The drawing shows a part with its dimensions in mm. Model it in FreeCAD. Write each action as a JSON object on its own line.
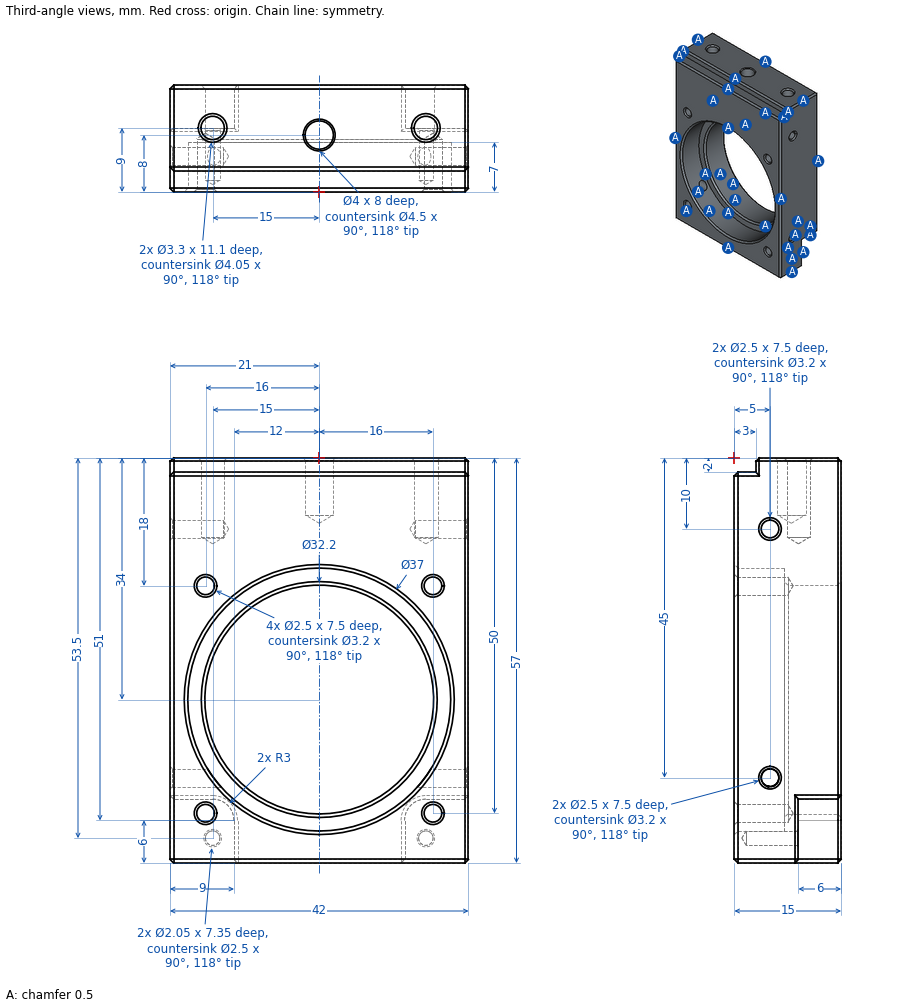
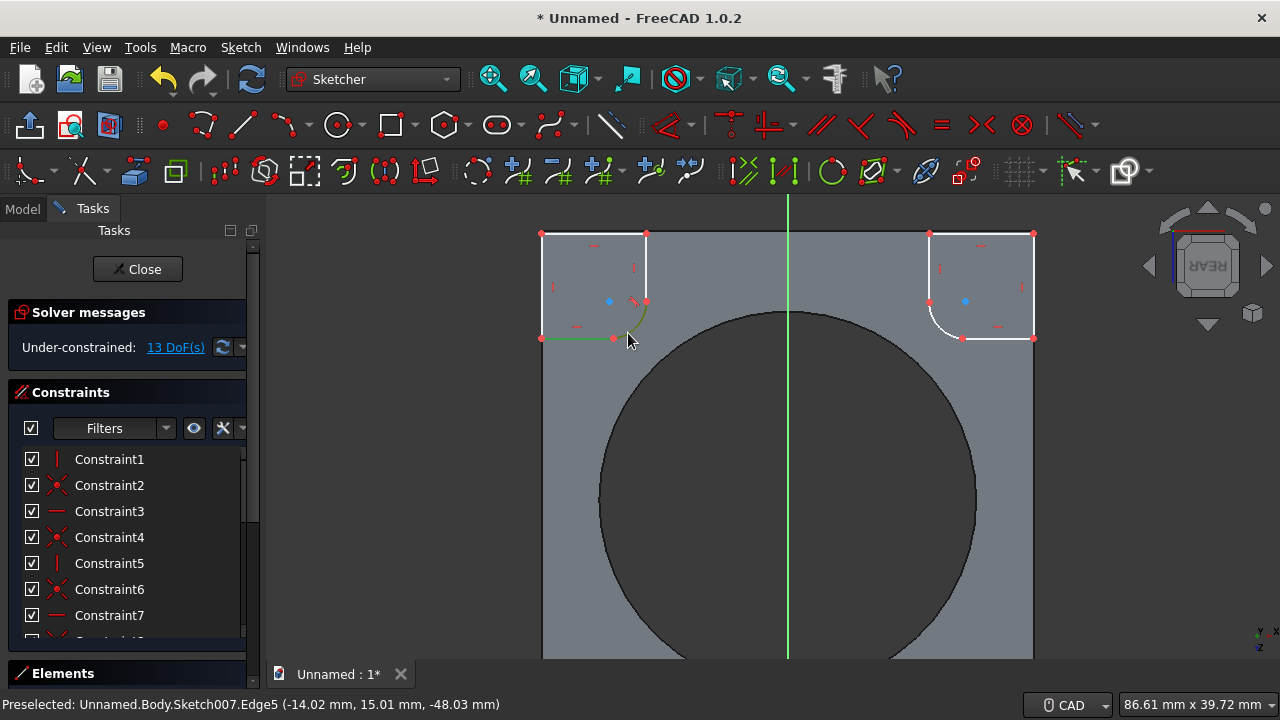
{"action": "left_click", "coordinate": [902, 126]}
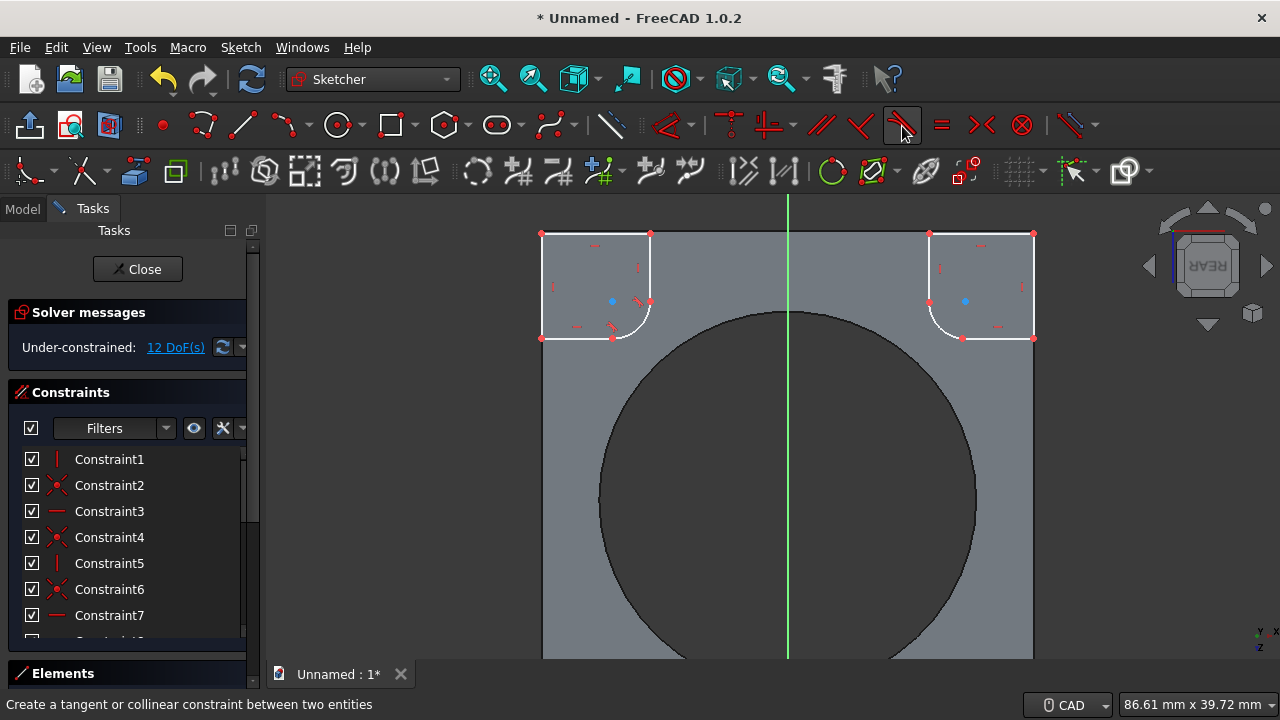
{"action": "left_click", "coordinate": [984, 339]}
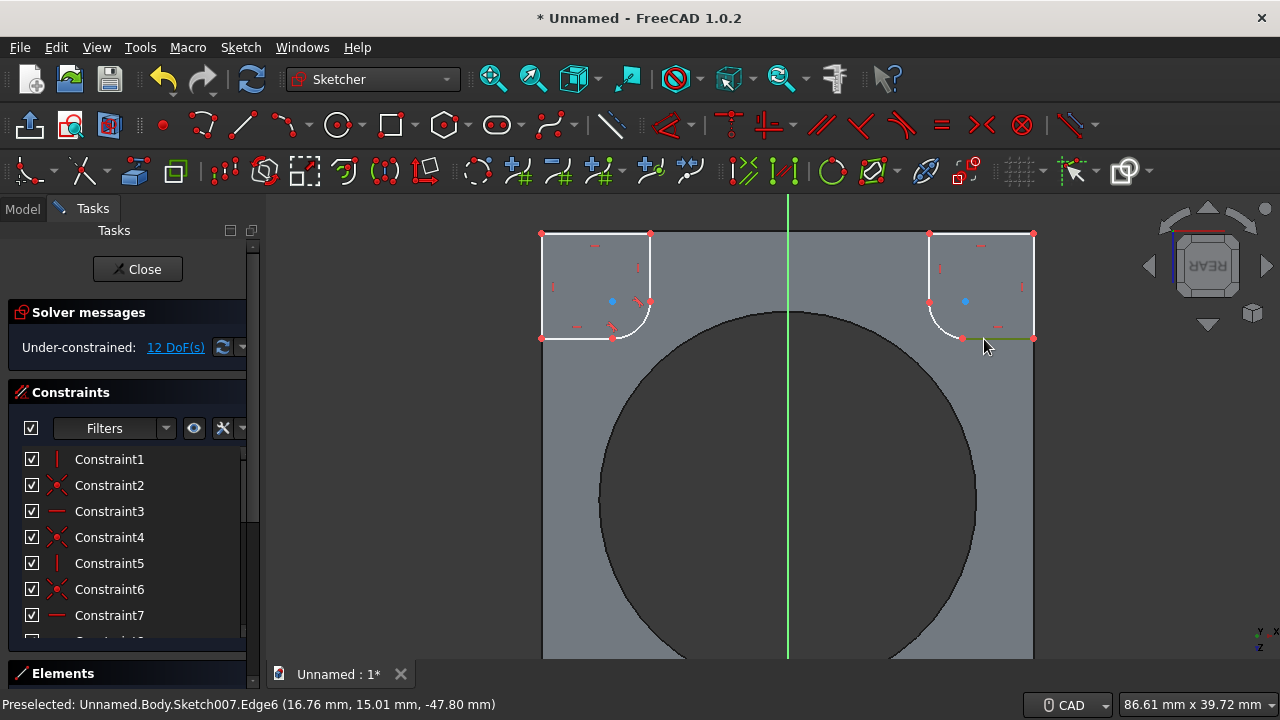
{"action": "left_click", "coordinate": [933, 318]}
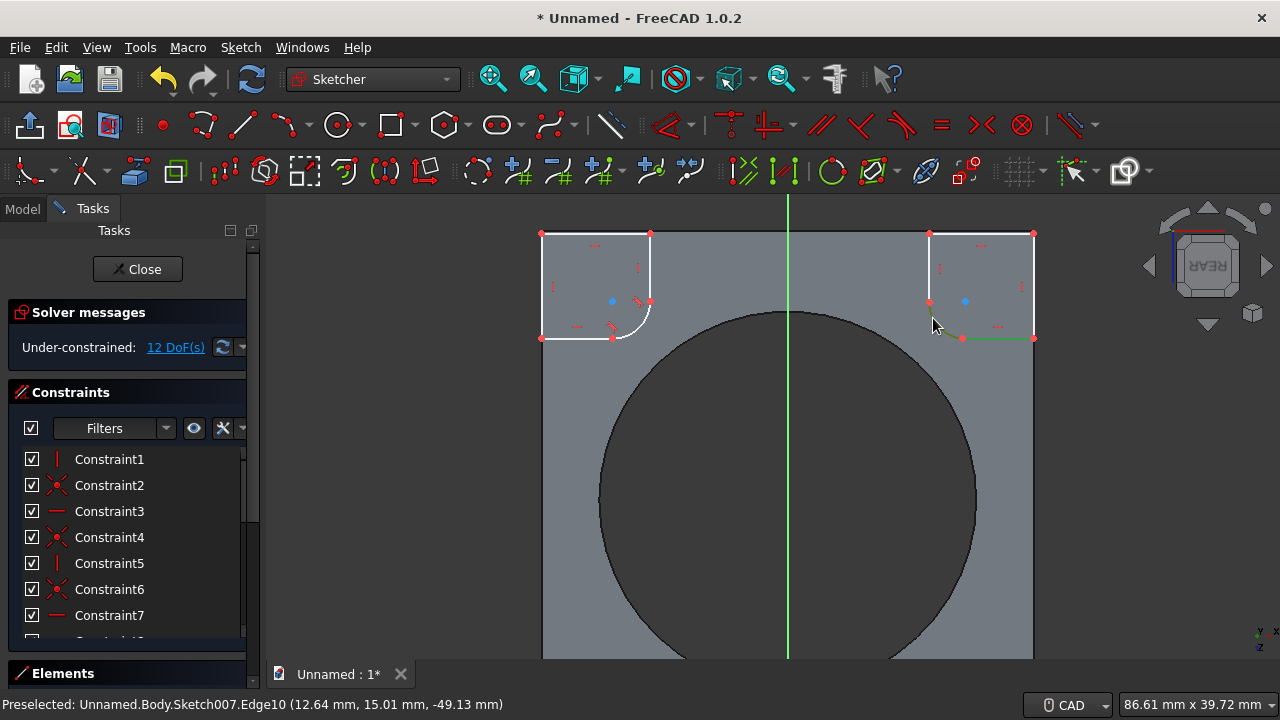
{"action": "key", "text": "t"}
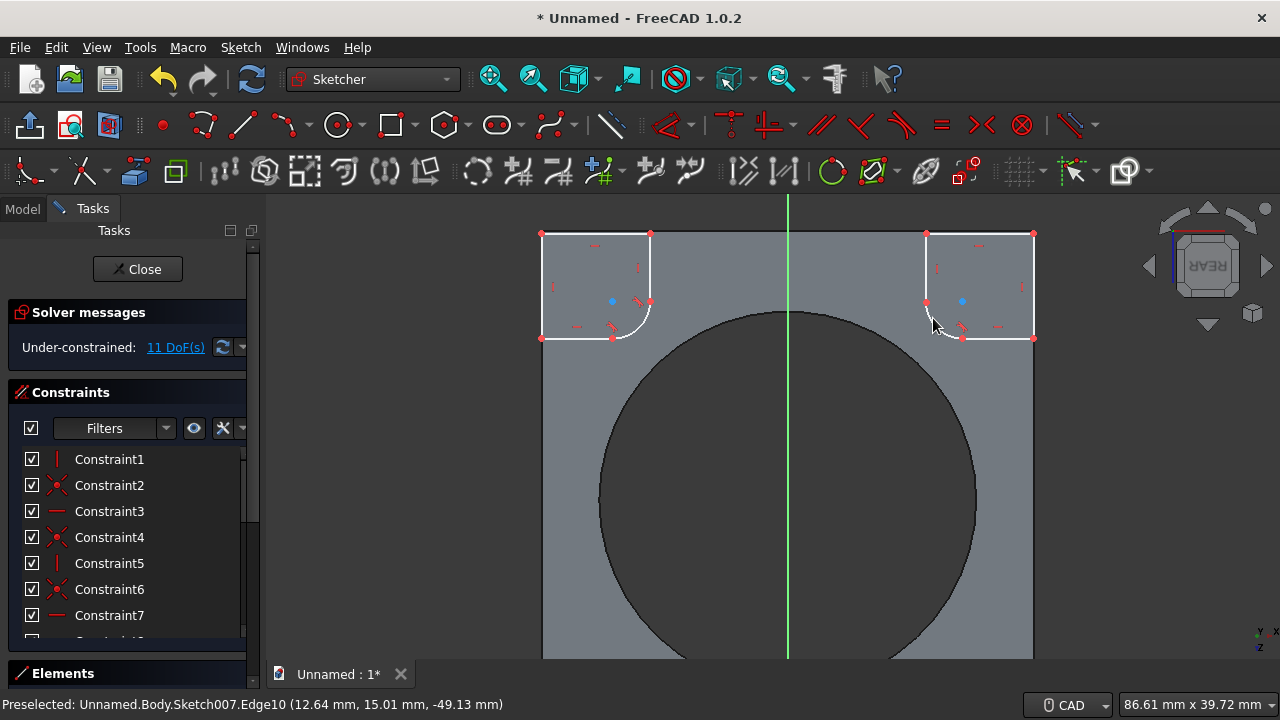
{"action": "left_click", "coordinate": [926, 255]}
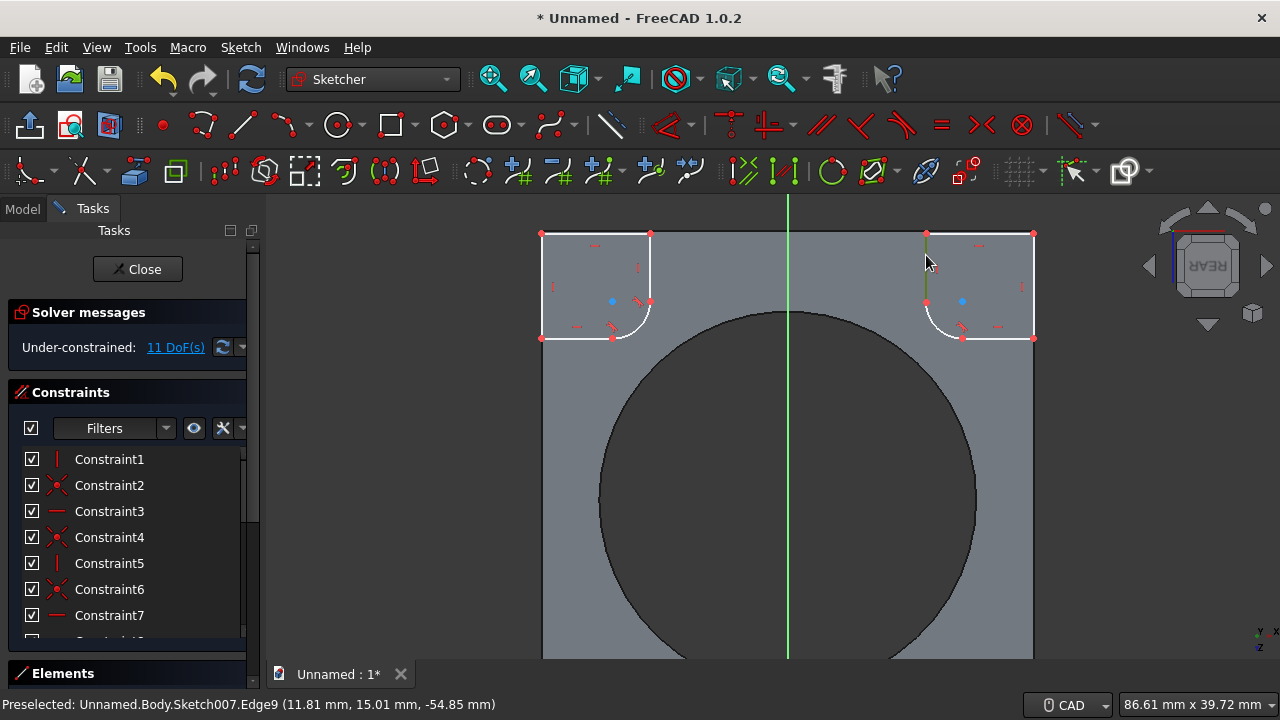
{"action": "left_click", "coordinate": [930, 319]}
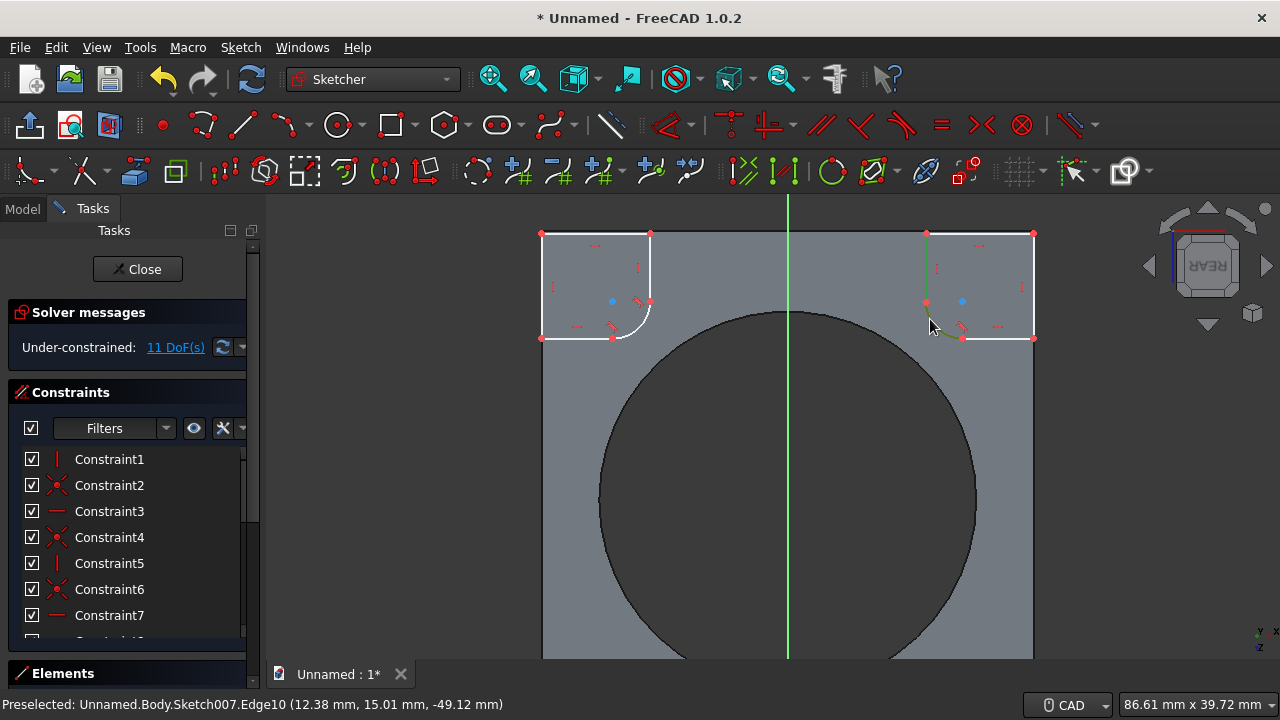
{"action": "left_click", "coordinate": [902, 126]}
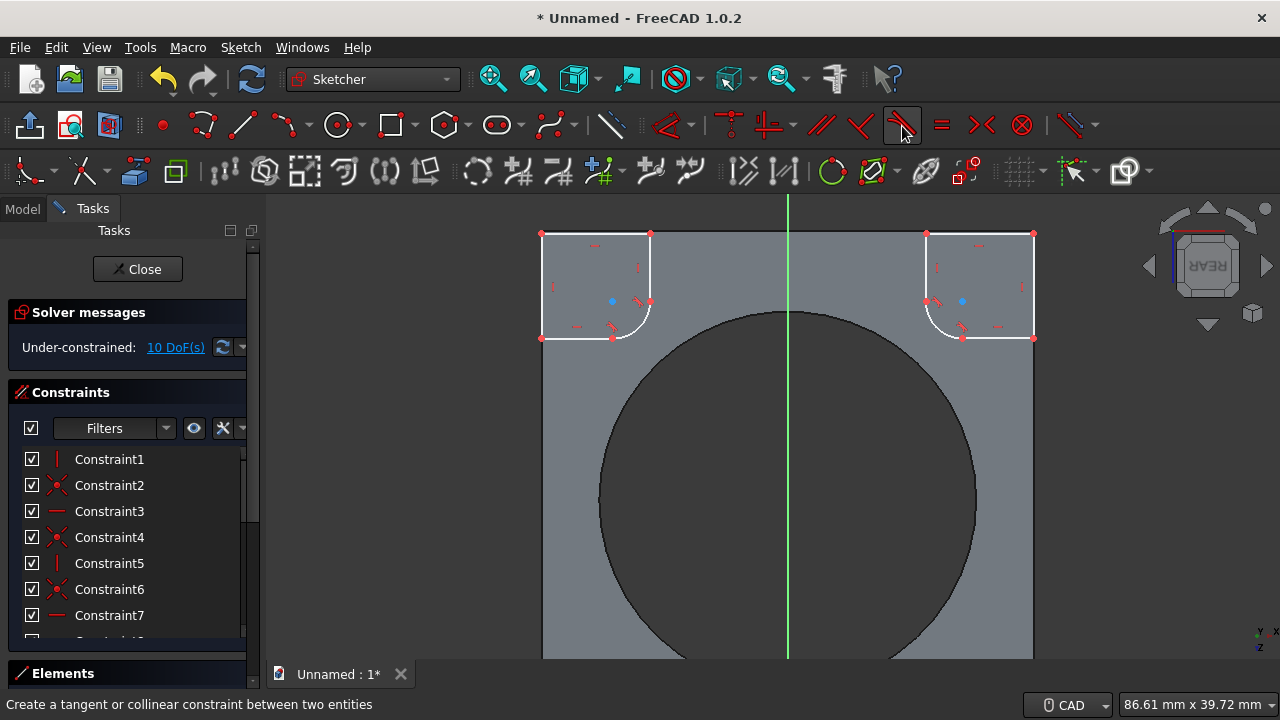
{"action": "left_click", "coordinate": [630, 335]}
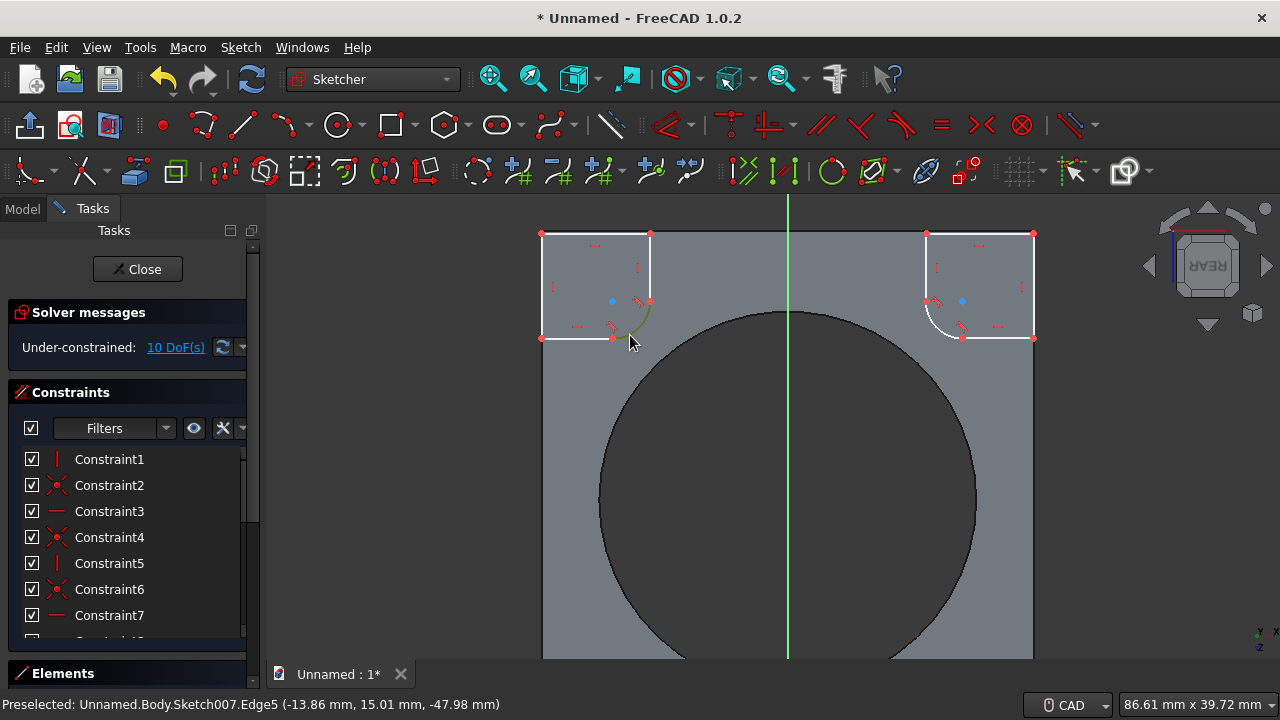
{"action": "left_click", "coordinate": [930, 318]}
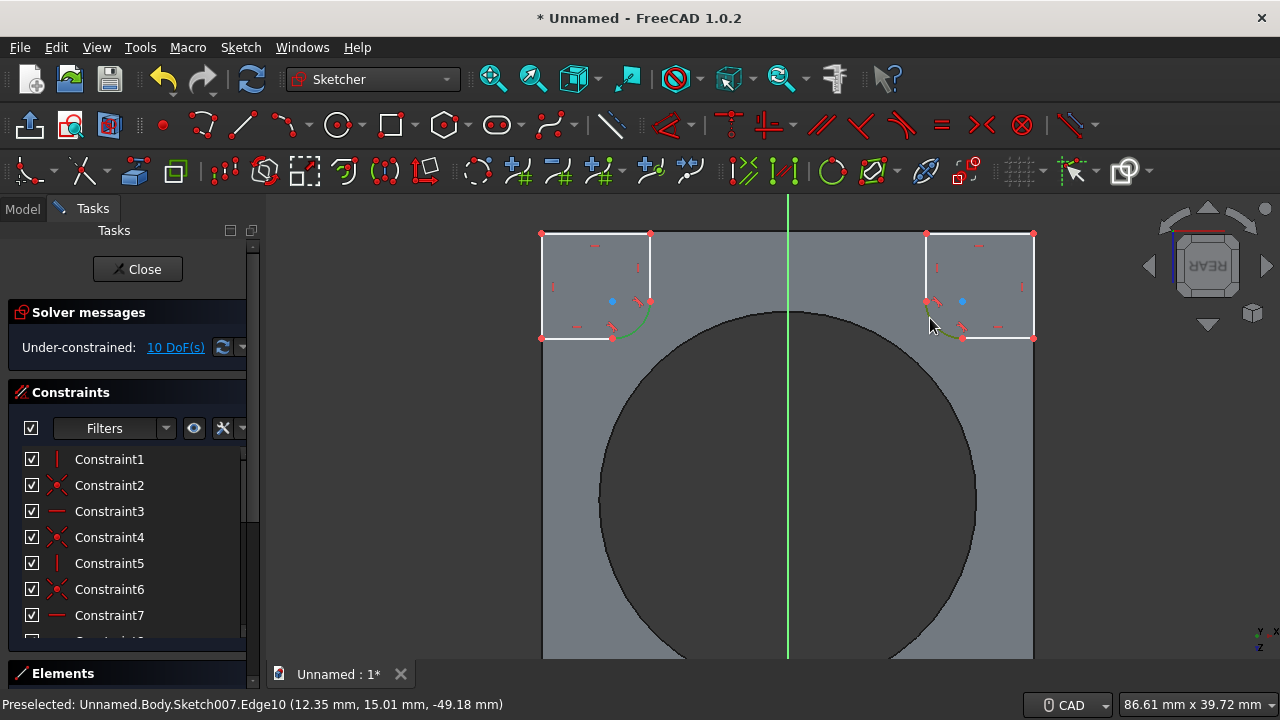
{"action": "key", "text": "e"}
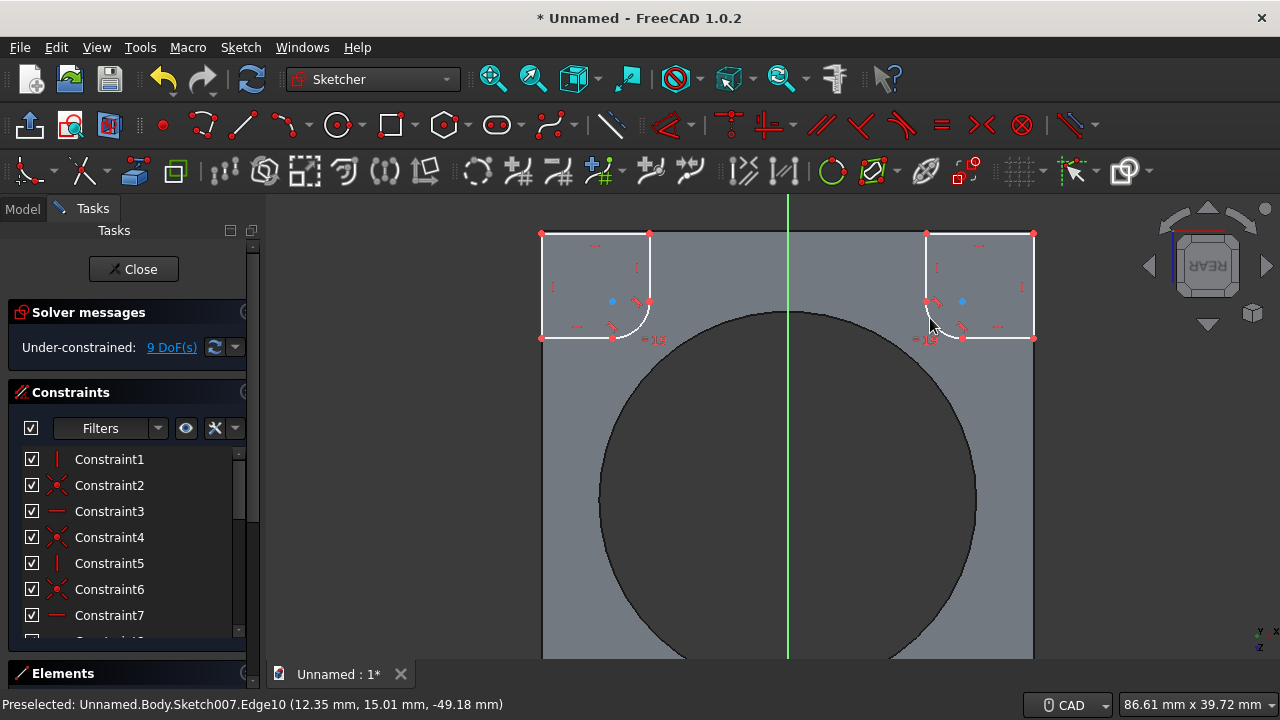
{"action": "left_click", "coordinate": [613, 301]}